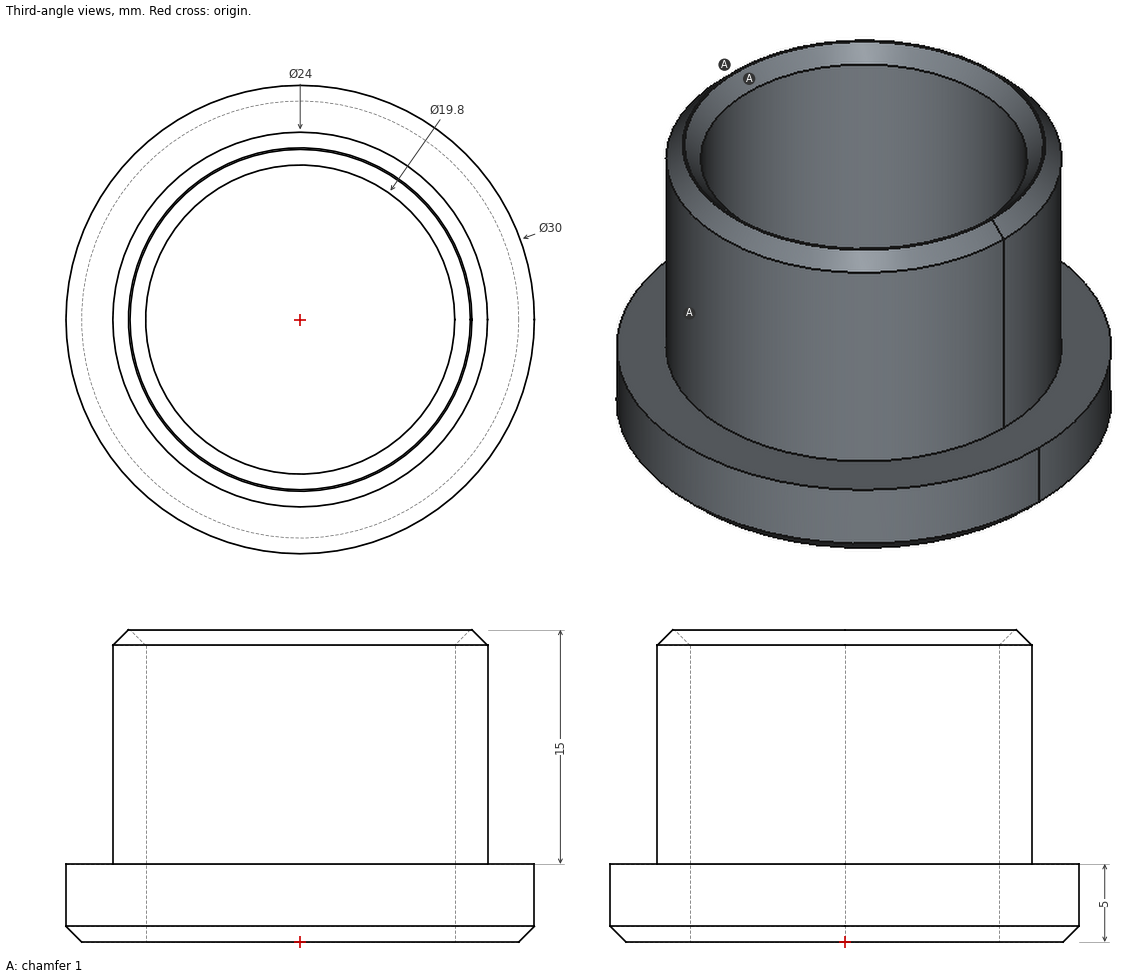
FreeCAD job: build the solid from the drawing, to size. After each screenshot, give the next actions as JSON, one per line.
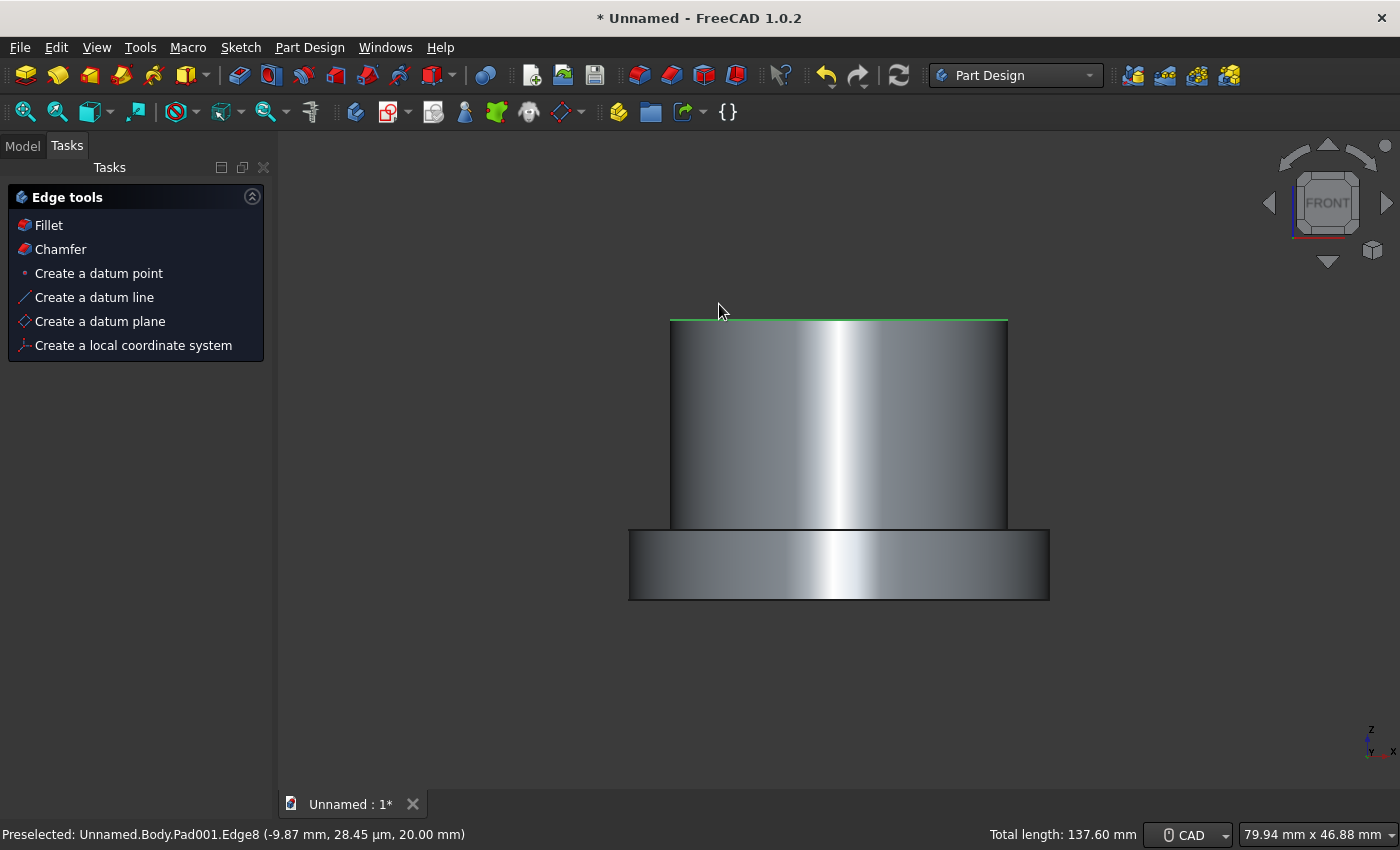
{"action": "left_click", "coordinate": [26, 112]}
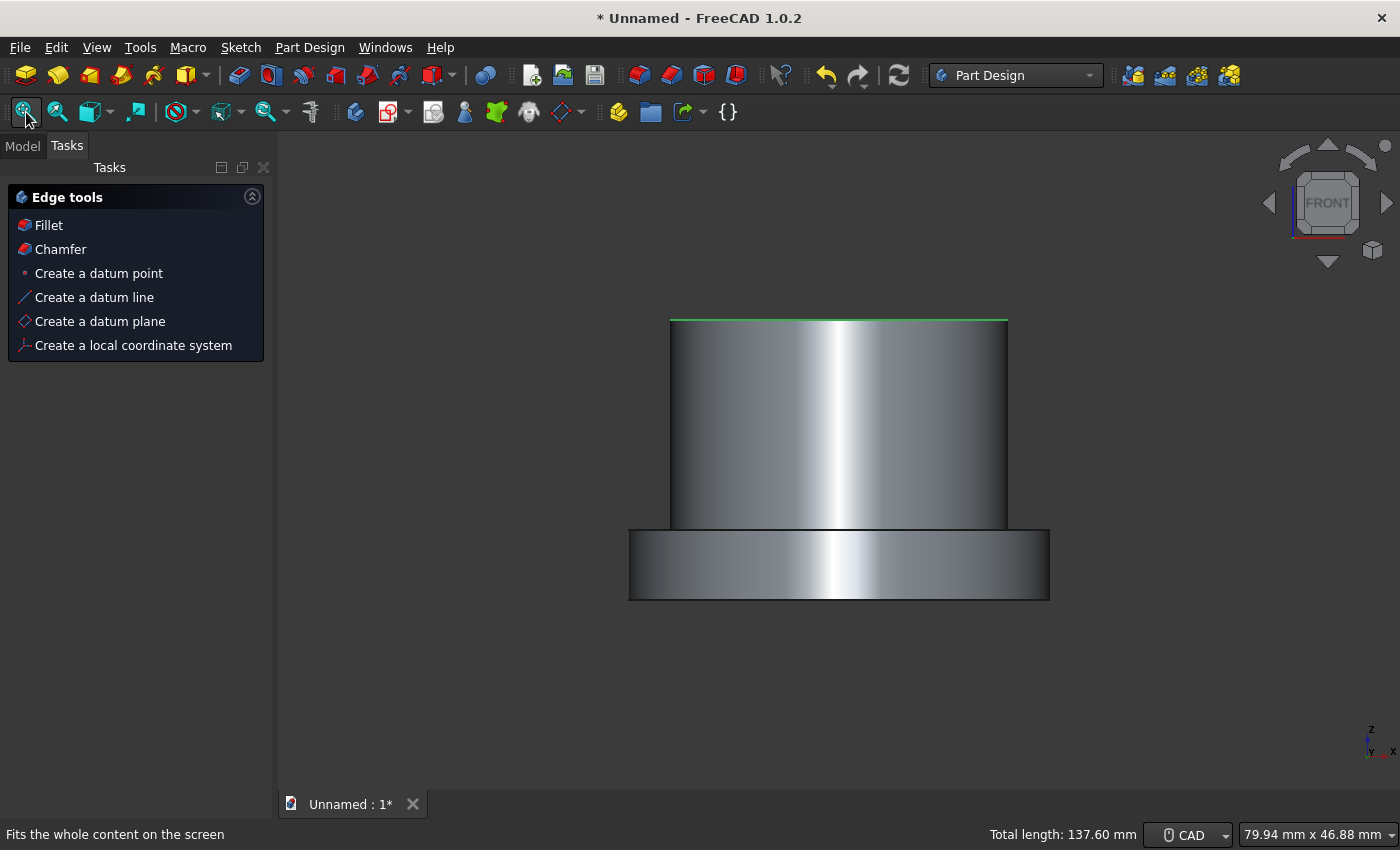
{"action": "left_click", "coordinate": [669, 599], "text": "ctrl"}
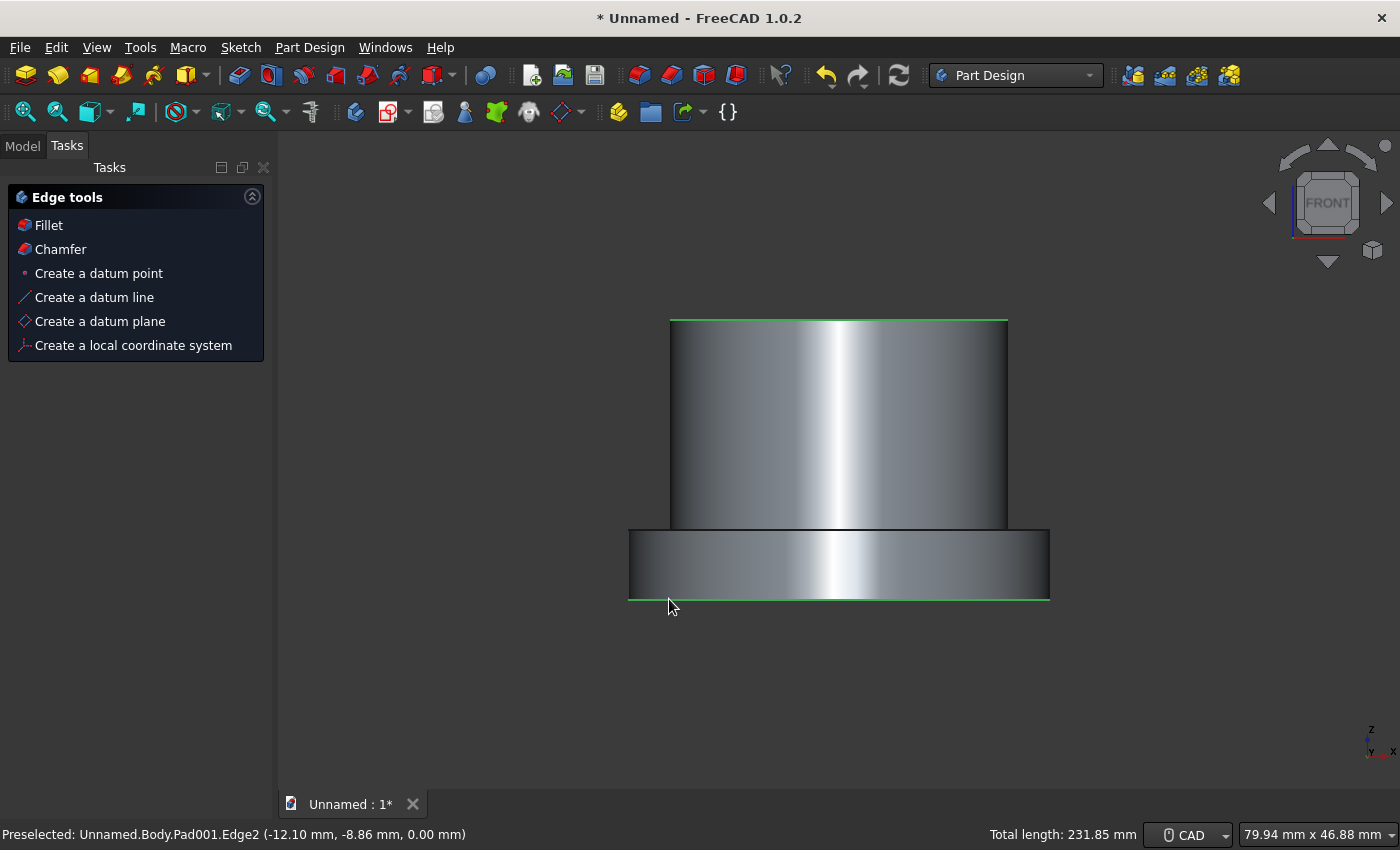
{"action": "left_click", "coordinate": [672, 76]}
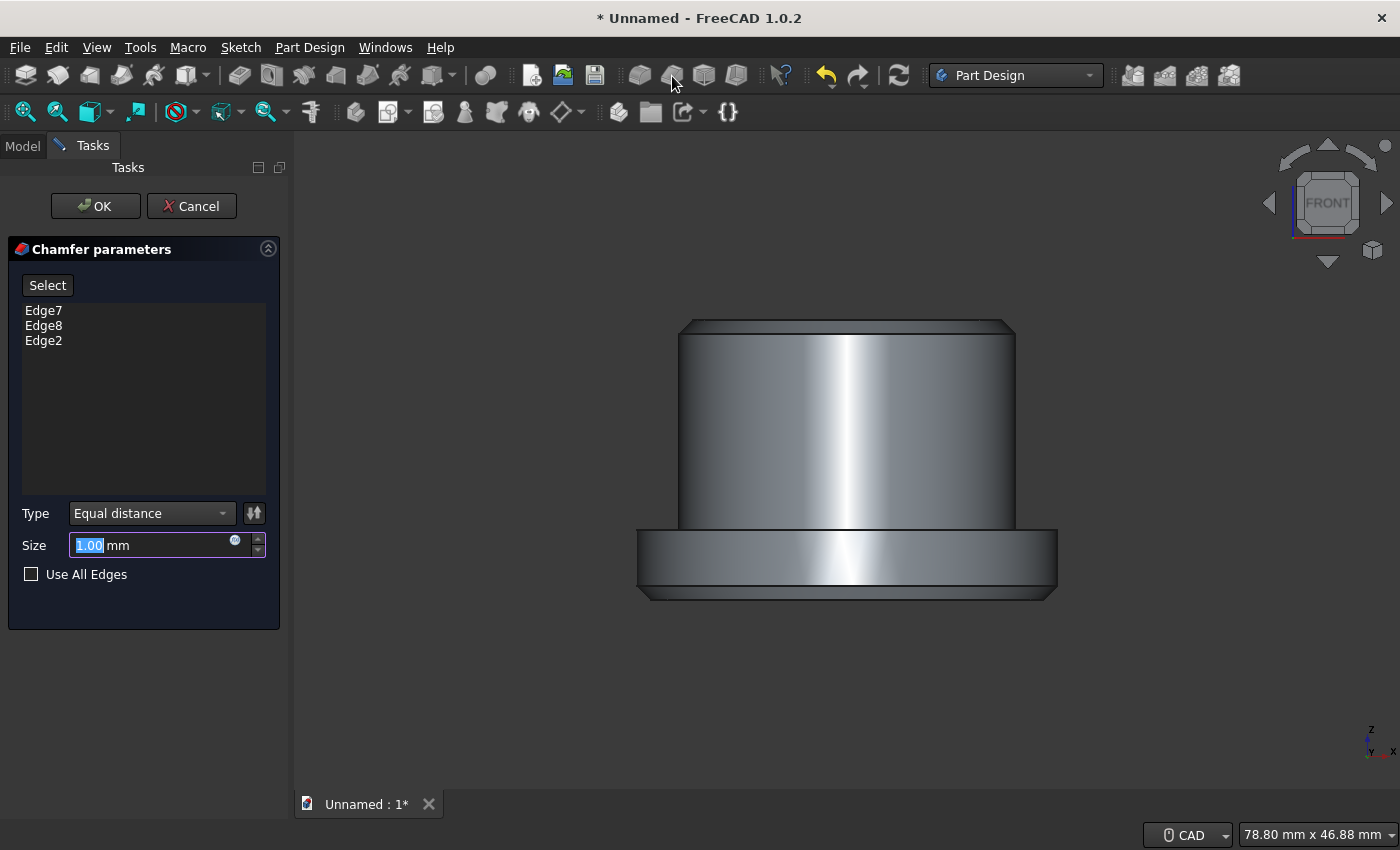
{"action": "type", "text": "1"}
{"action": "key", "text": "Tab"}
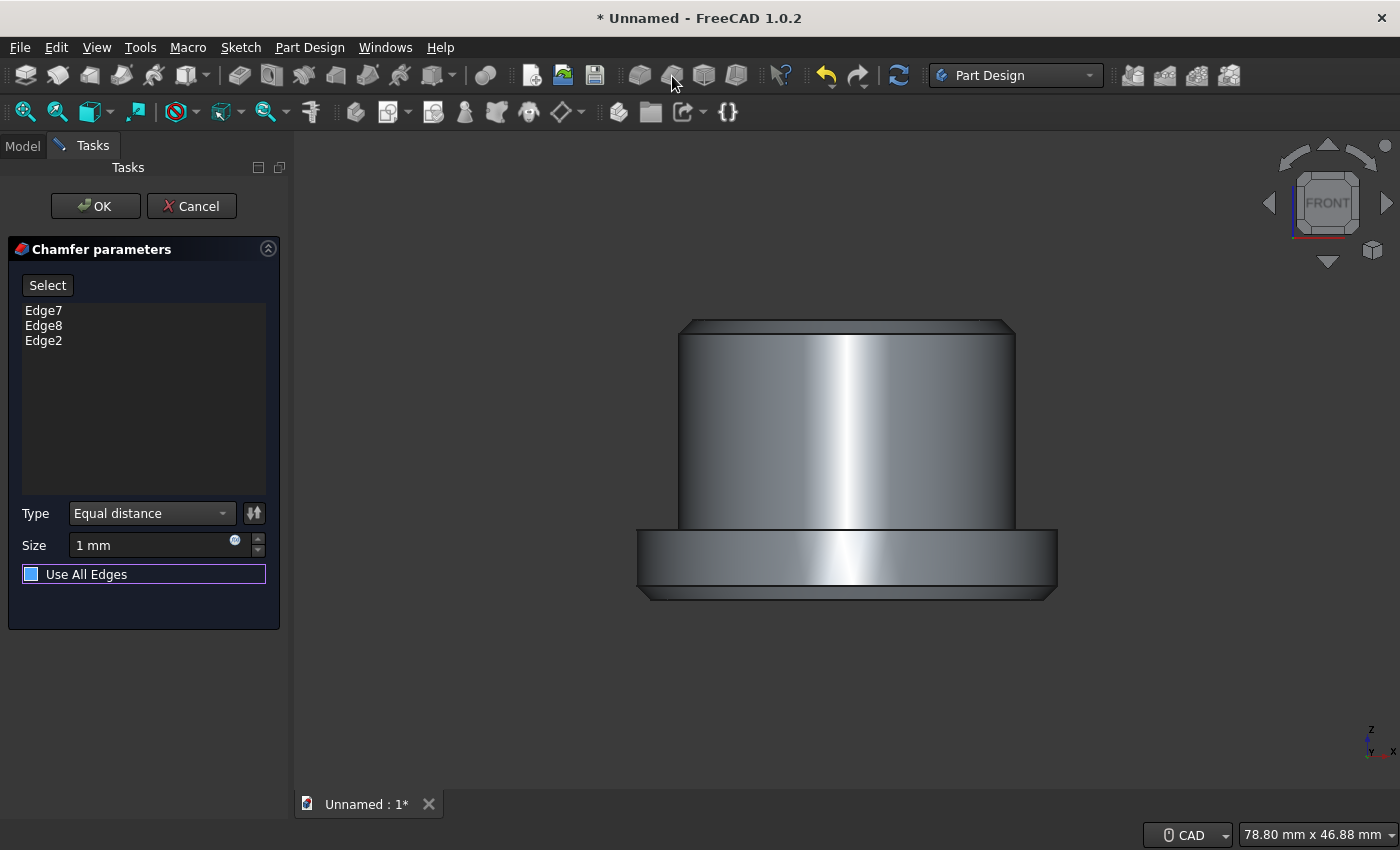
{"action": "left_click", "coordinate": [96, 206]}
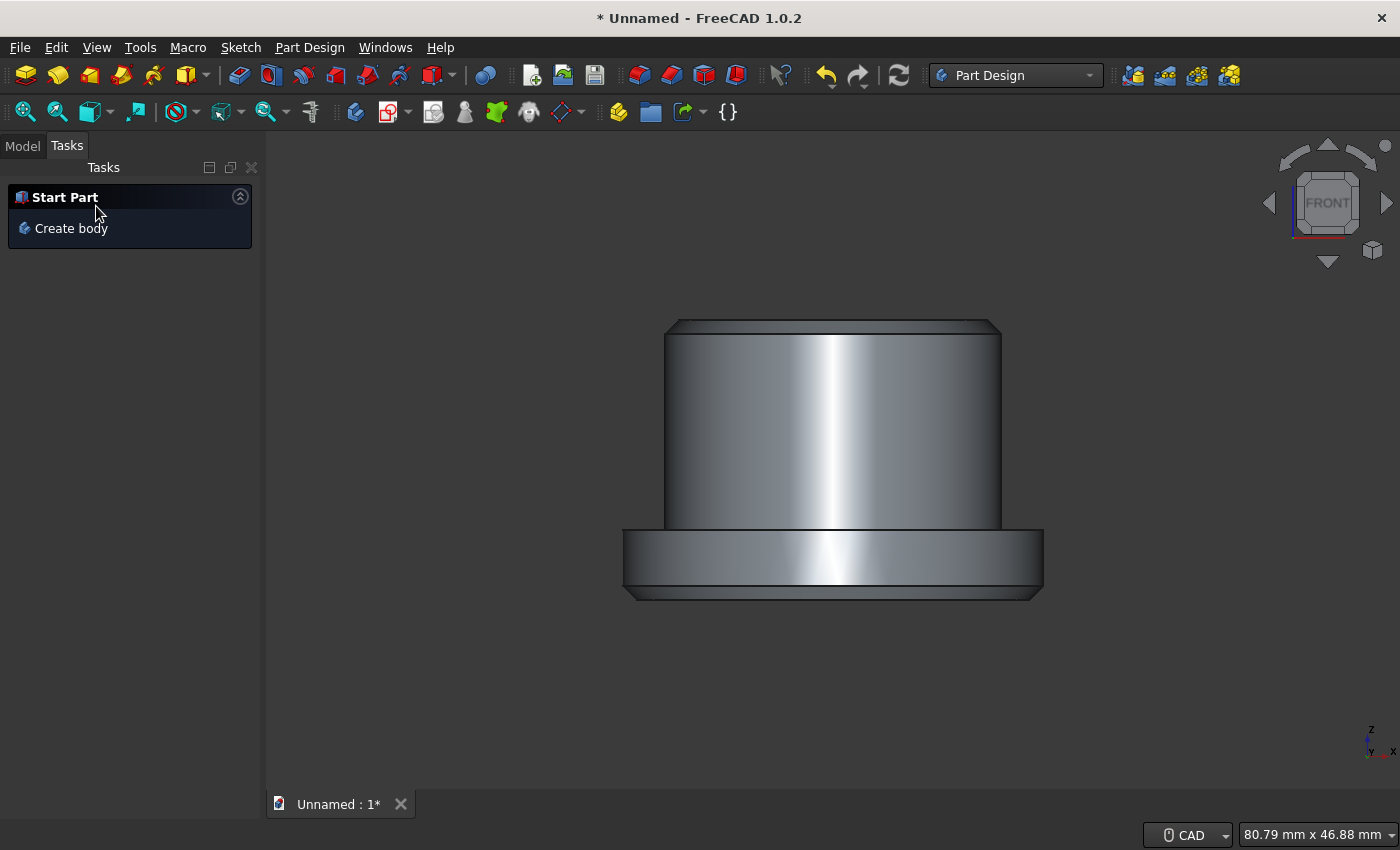
{"action": "key", "text": "0"}